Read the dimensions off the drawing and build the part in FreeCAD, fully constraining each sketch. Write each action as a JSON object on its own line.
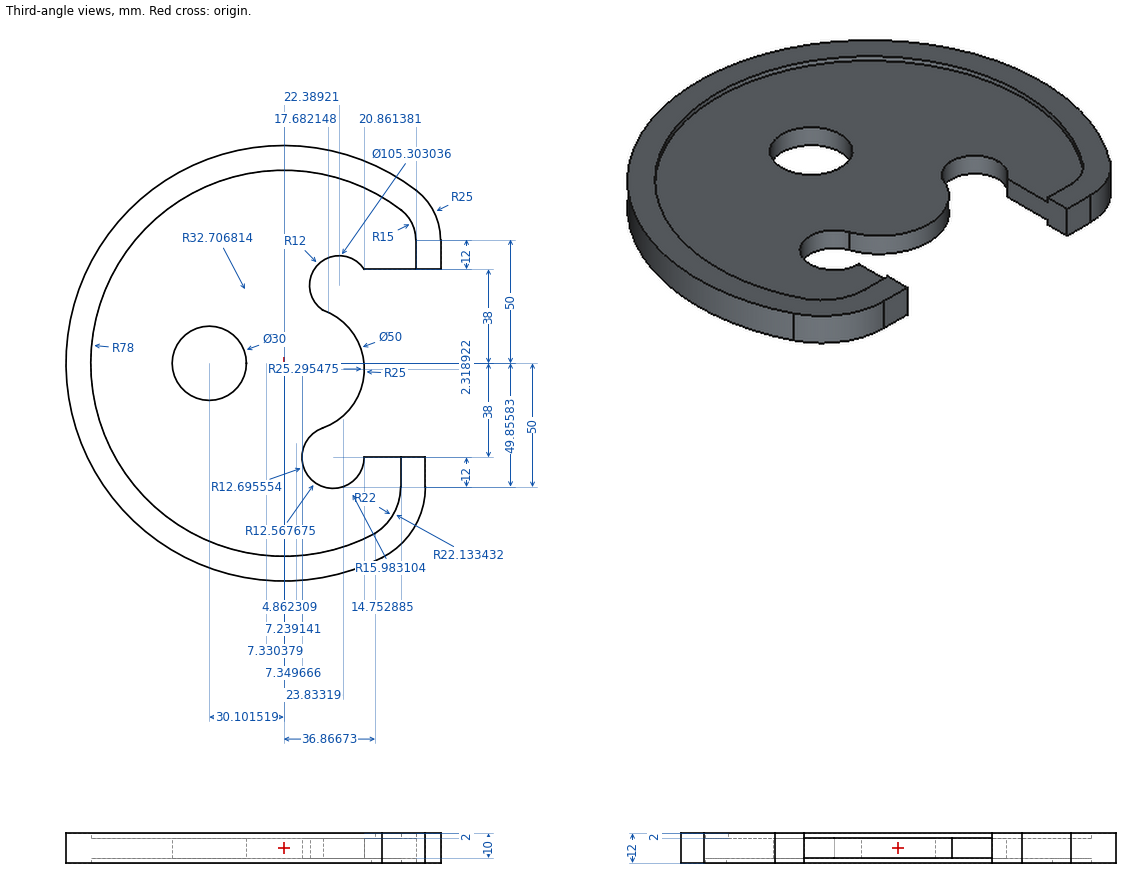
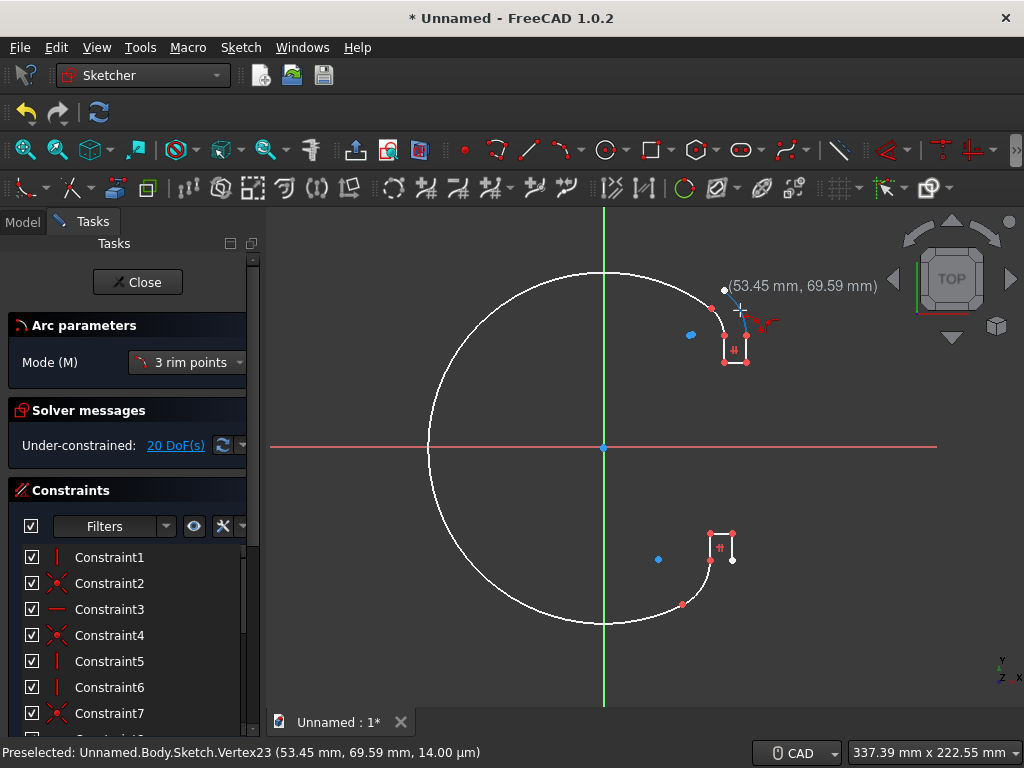
{"action": "left_click", "coordinate": [693, 624]}
{"action": "left_click", "coordinate": [407, 429]}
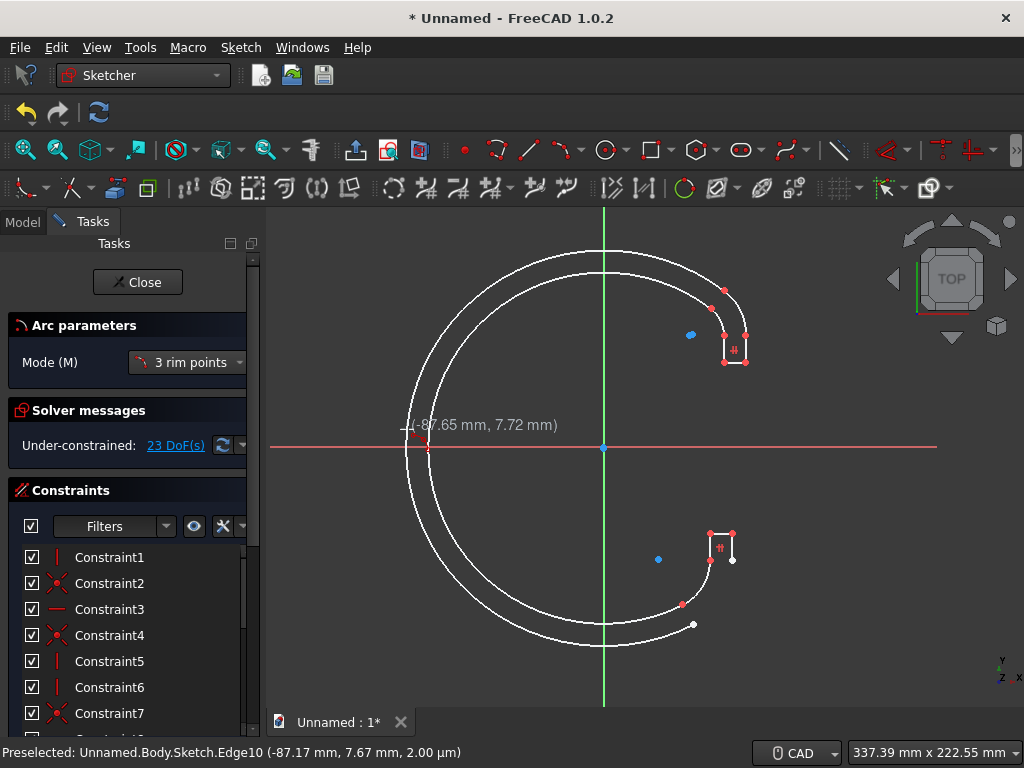
{"action": "left_click", "coordinate": [693, 625]}
{"action": "left_click", "coordinate": [732, 561]}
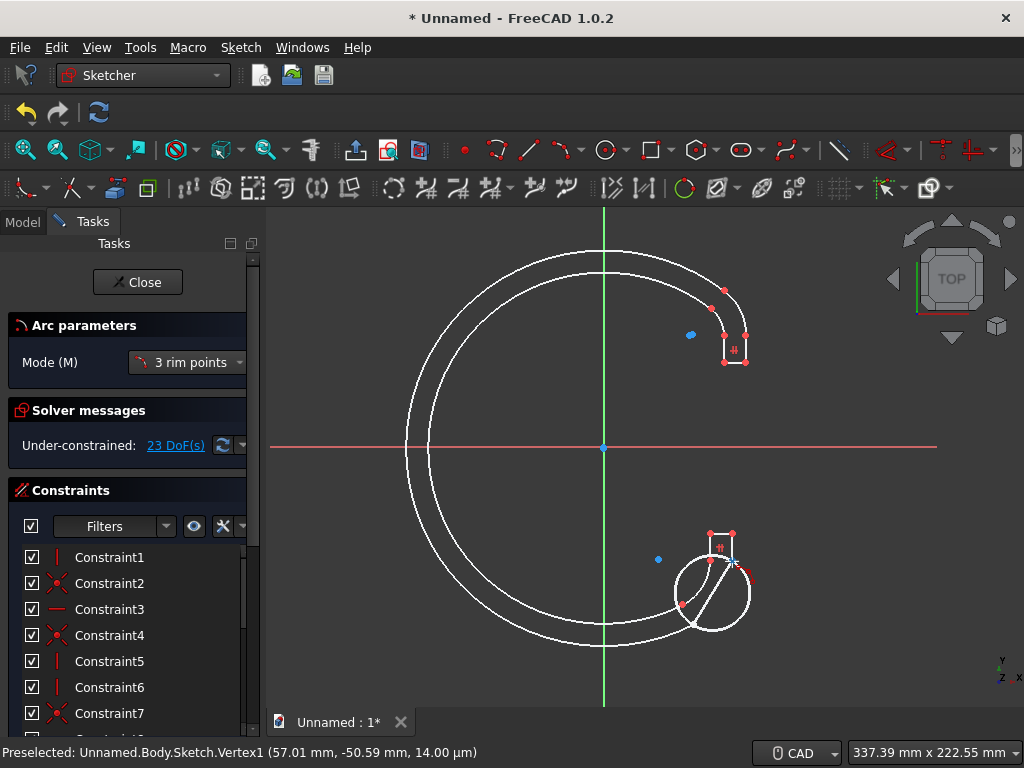
{"action": "scroll", "coordinate": [722, 597], "scroll_direction": "up", "scroll_amount": 2}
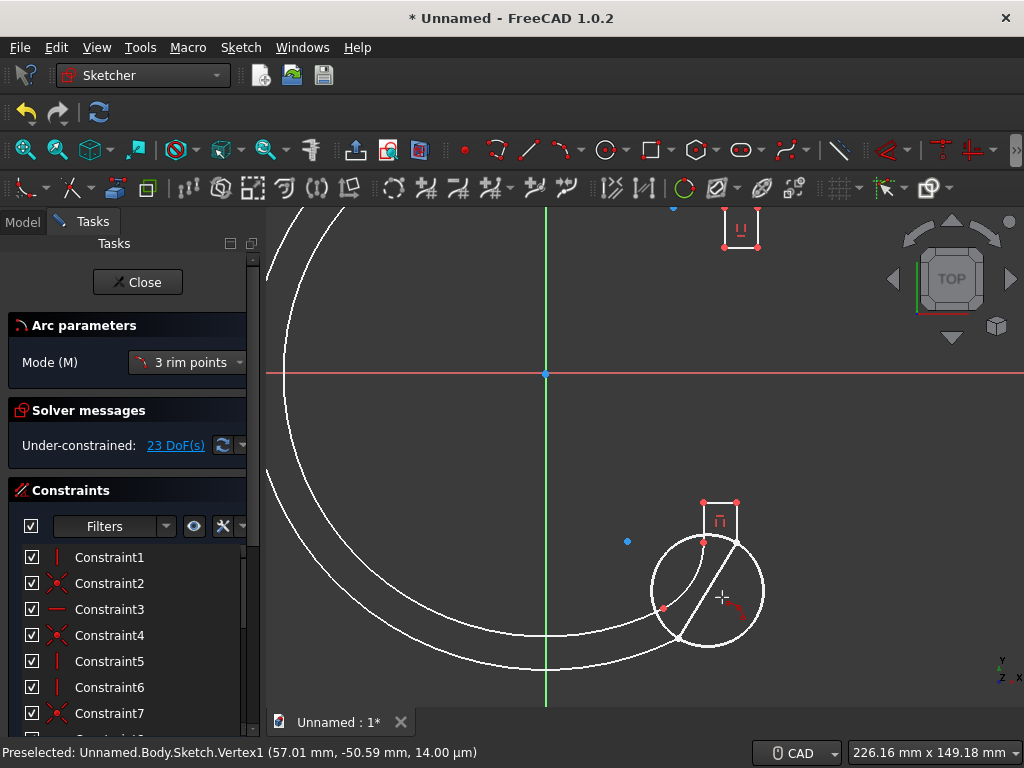
{"action": "left_click", "coordinate": [721, 597]}
{"action": "key", "text": "Escape"}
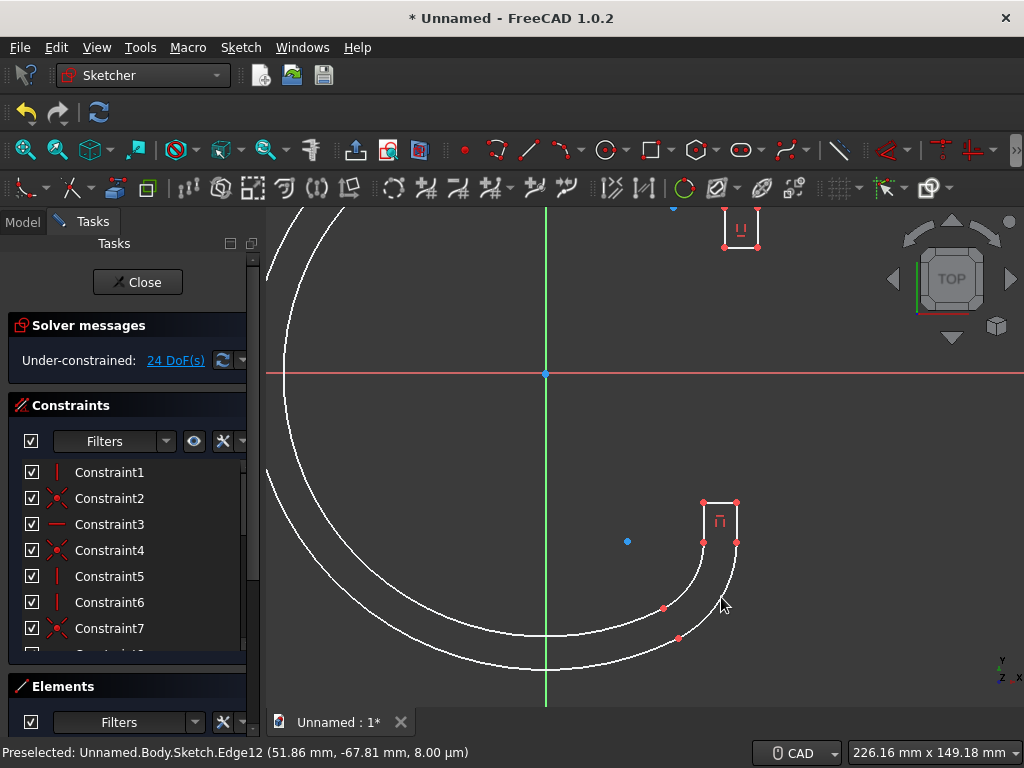
{"action": "left_click", "coordinate": [737, 531]}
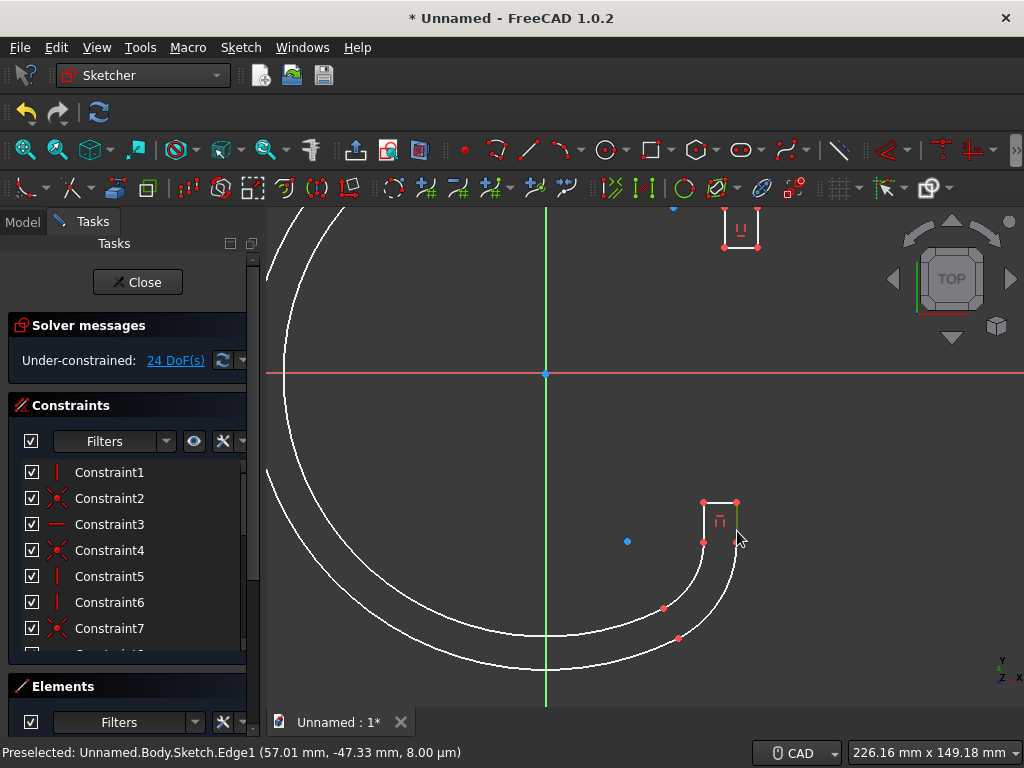
{"action": "left_click", "coordinate": [706, 617]}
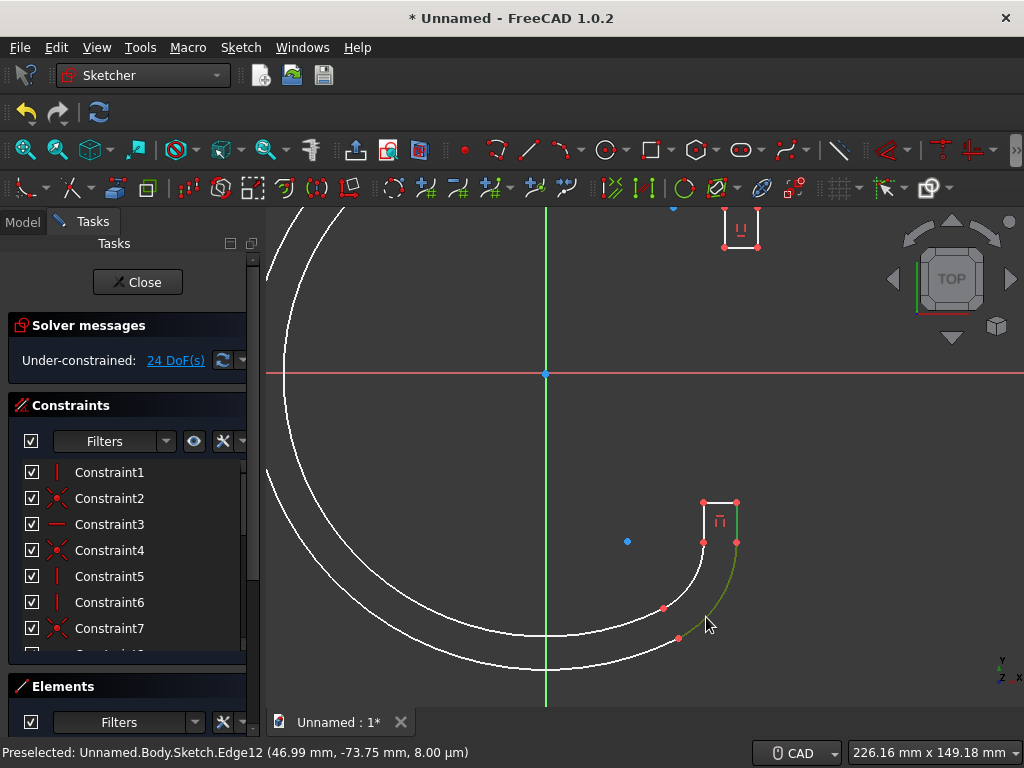
{"action": "key", "text": "t"}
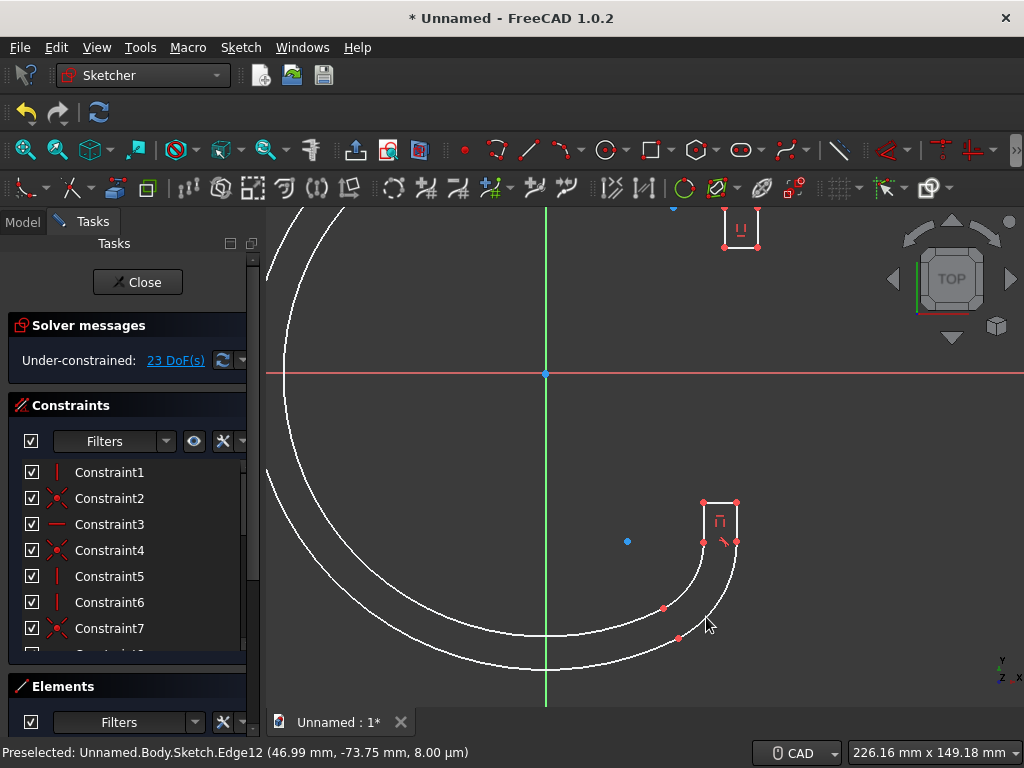
{"action": "left_click", "coordinate": [704, 515]}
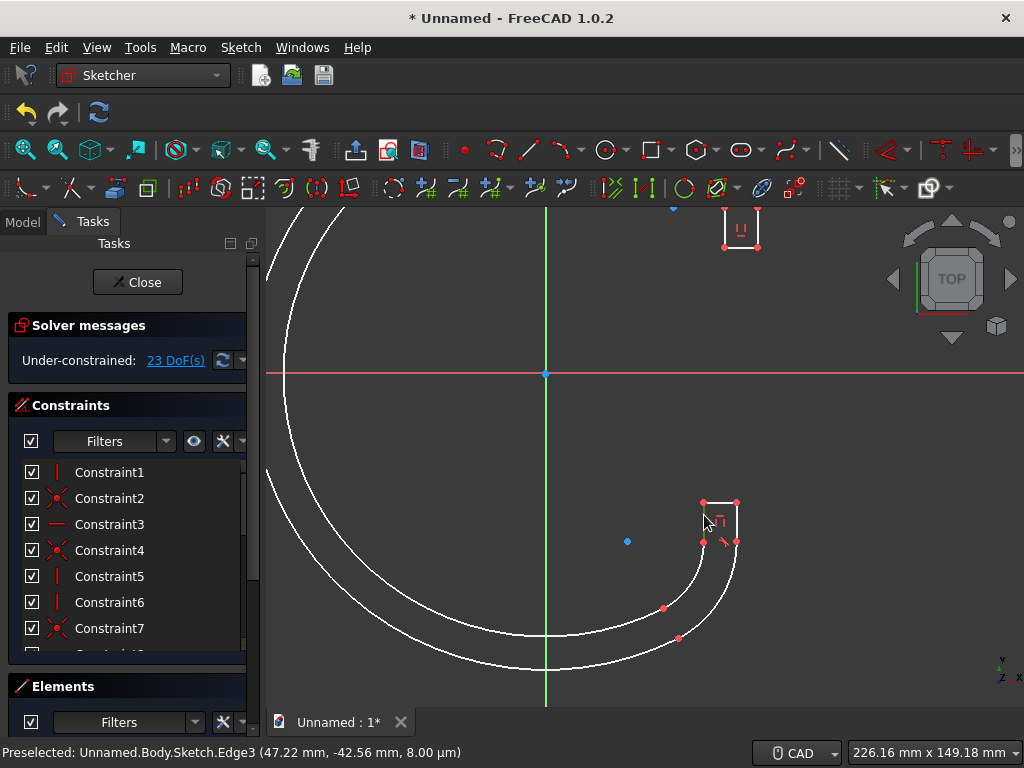
{"action": "left_click", "coordinate": [683, 594]}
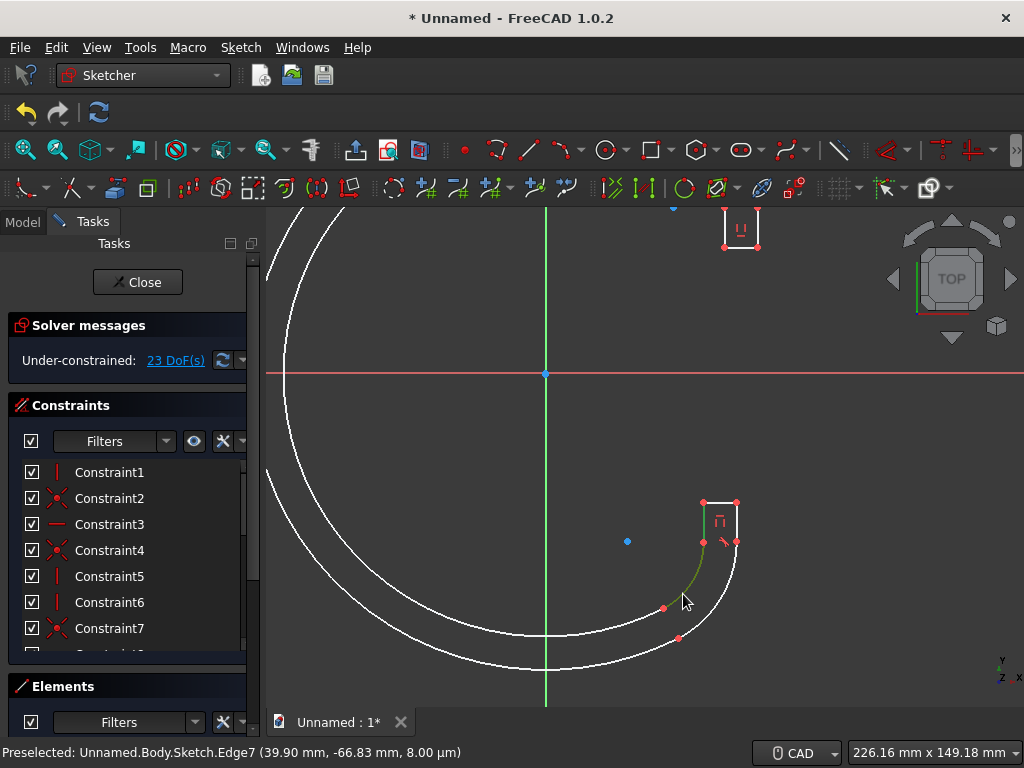
{"action": "key", "text": "t"}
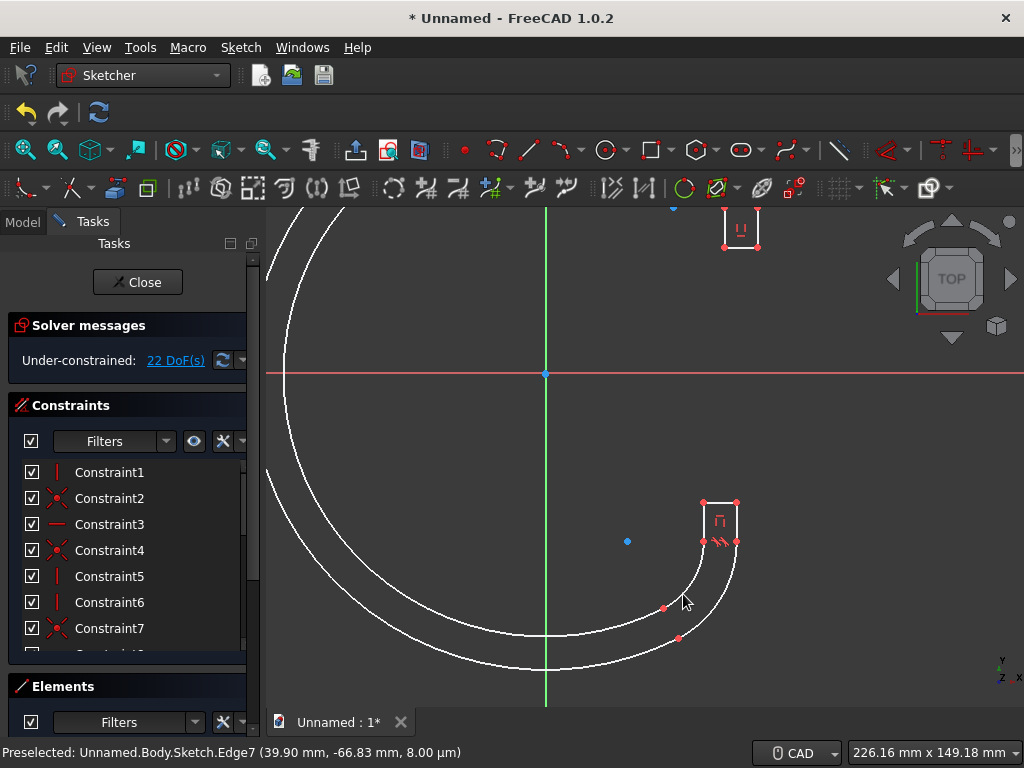
{"action": "left_click", "coordinate": [725, 235]}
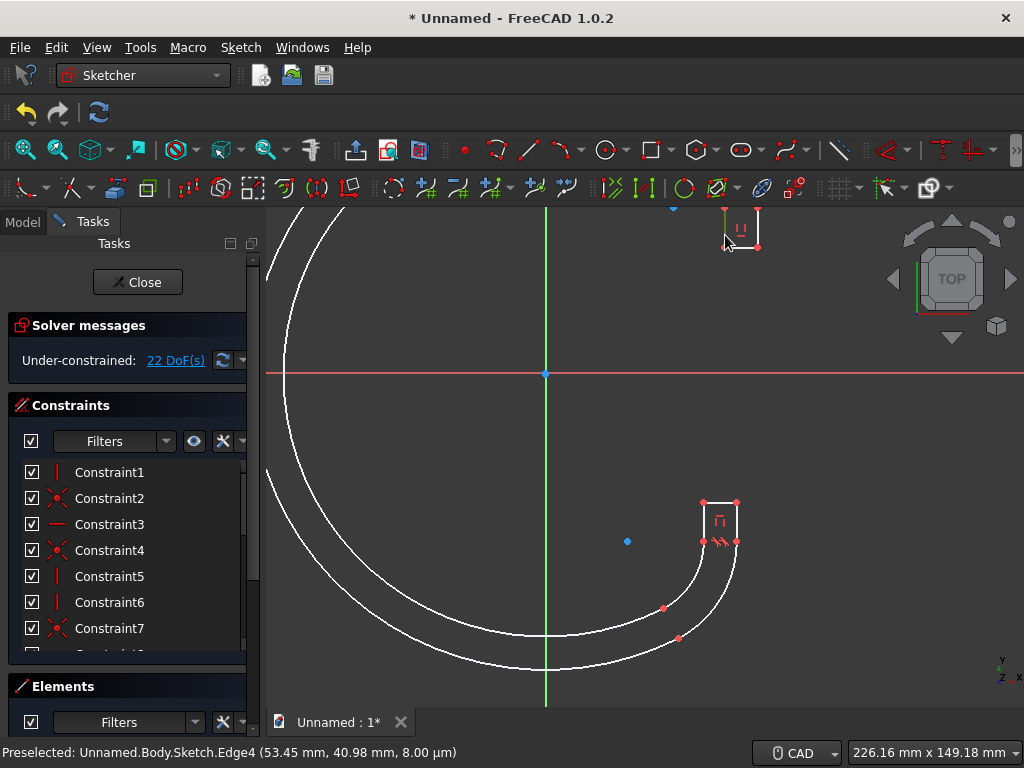
{"action": "scroll", "coordinate": [722, 597], "scroll_direction": "down", "scroll_amount": 2}